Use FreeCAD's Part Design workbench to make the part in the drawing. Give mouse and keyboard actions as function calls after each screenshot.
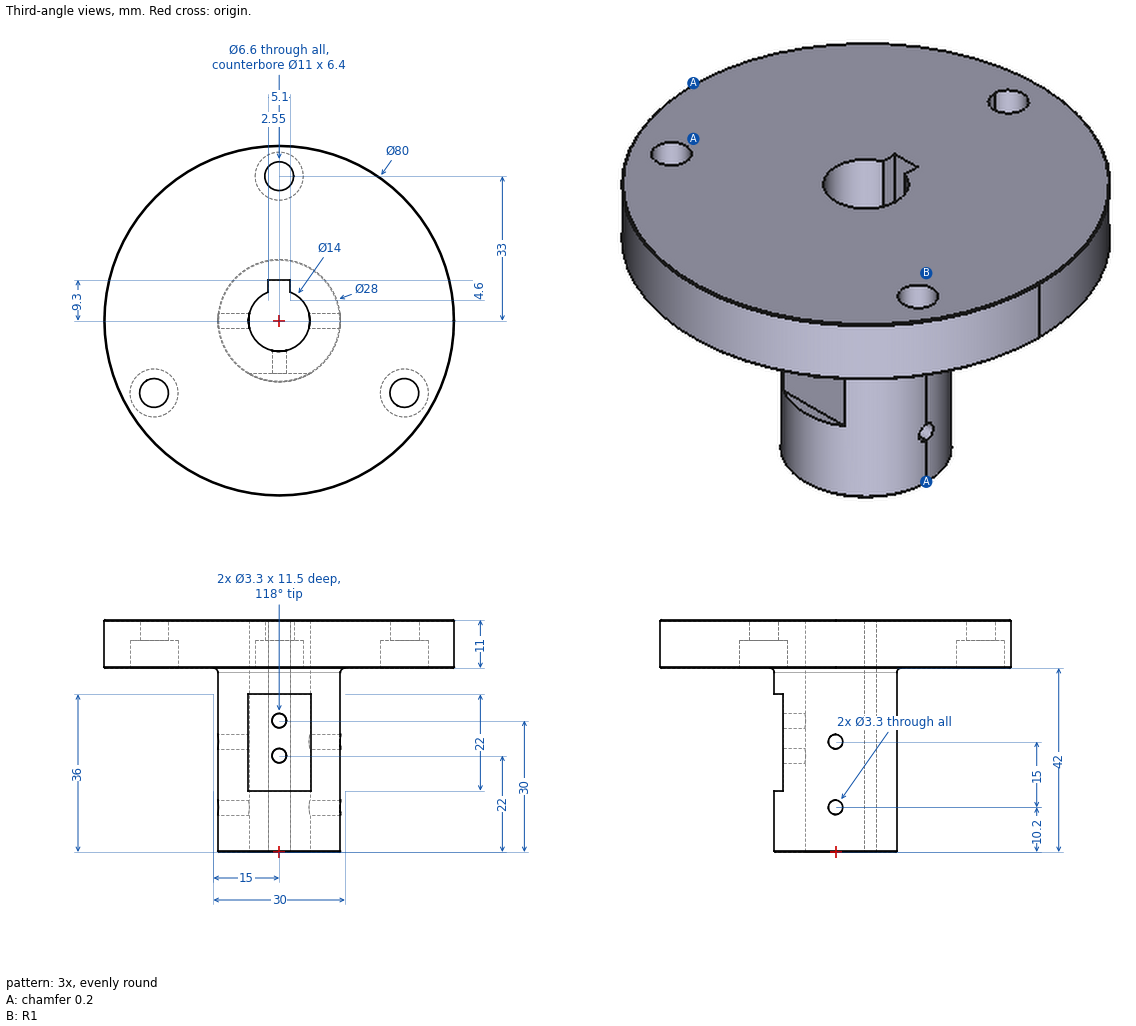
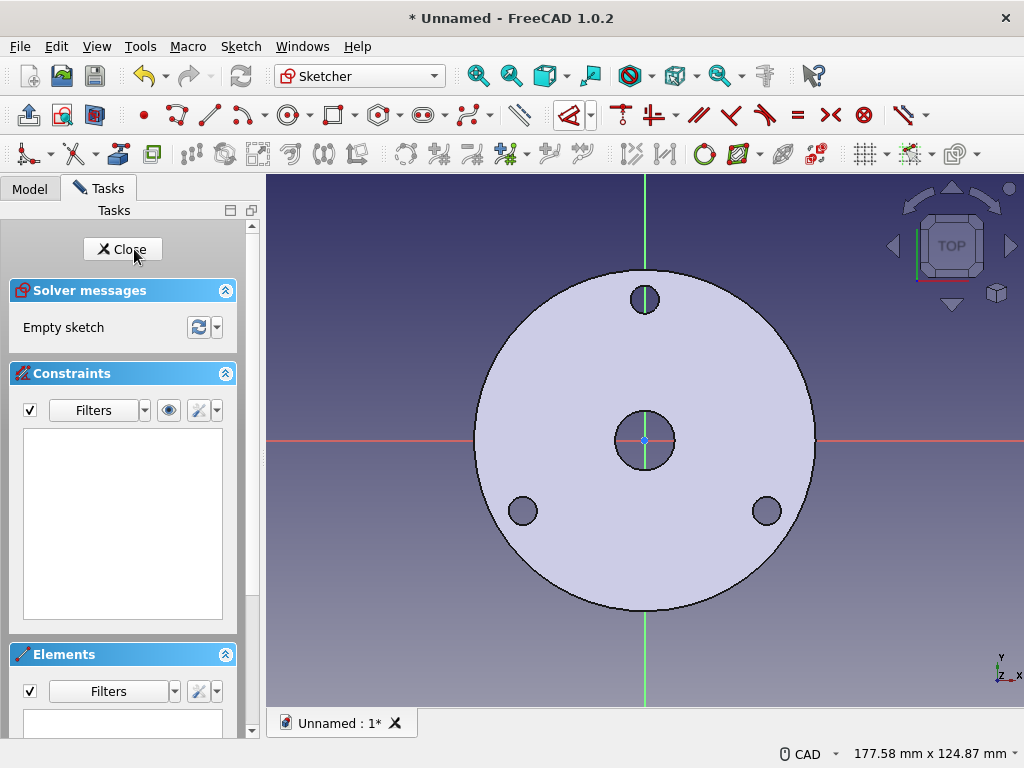
key(q)
key(s)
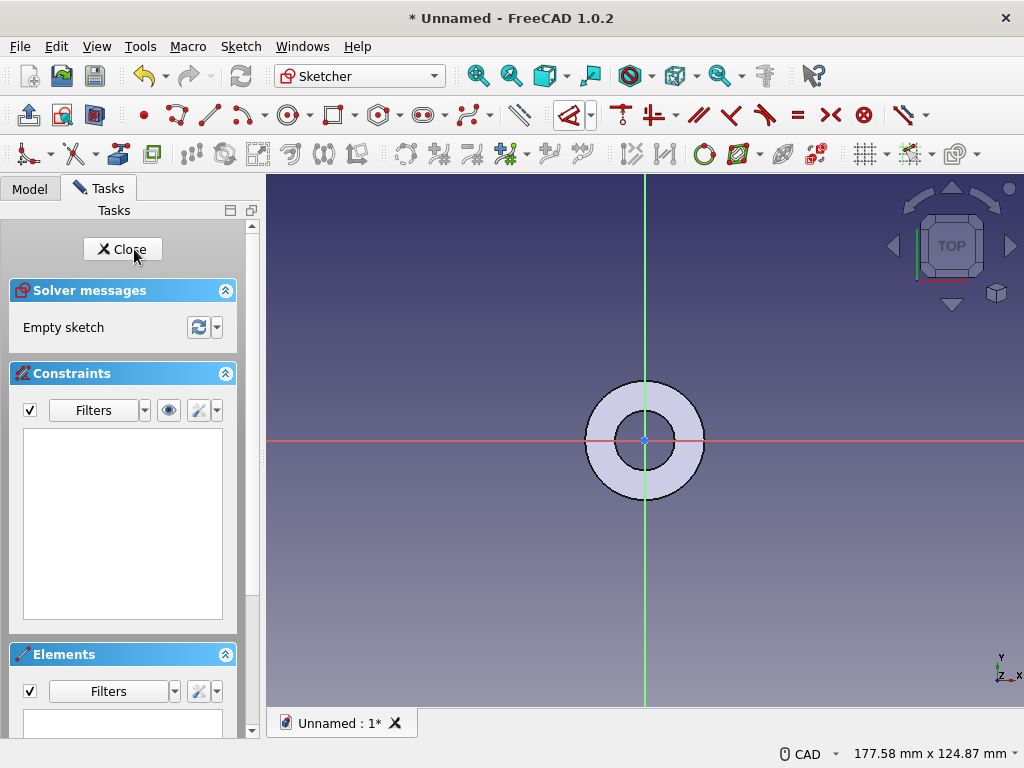
scroll(653, 418, up, 11)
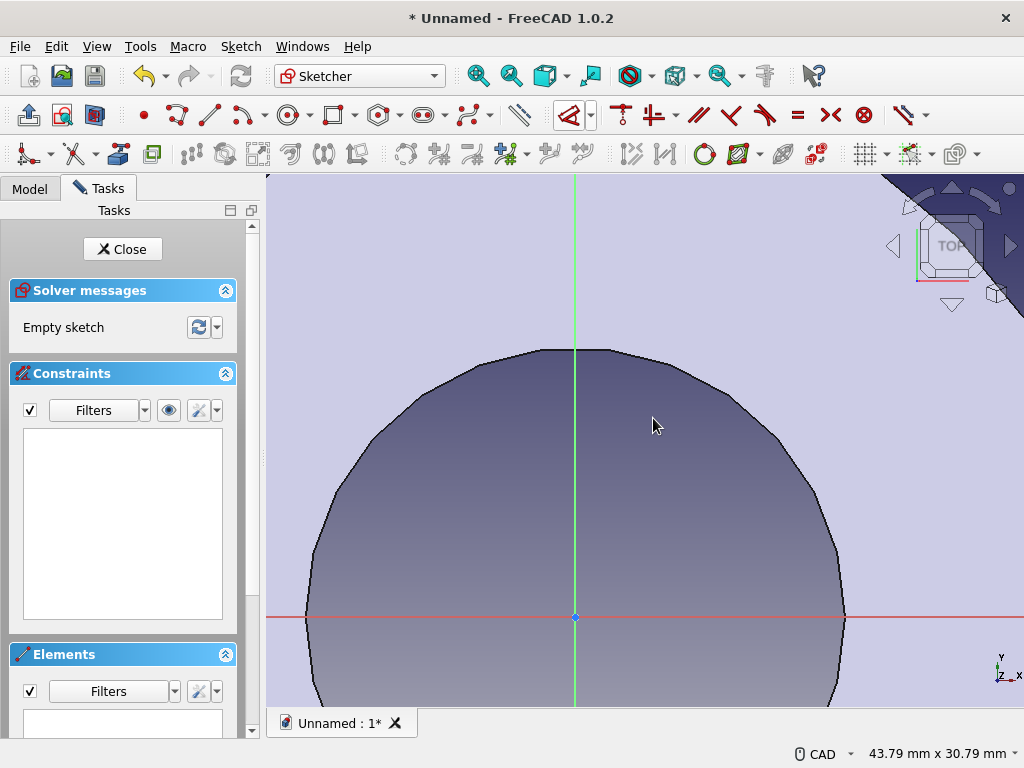
click(332, 116)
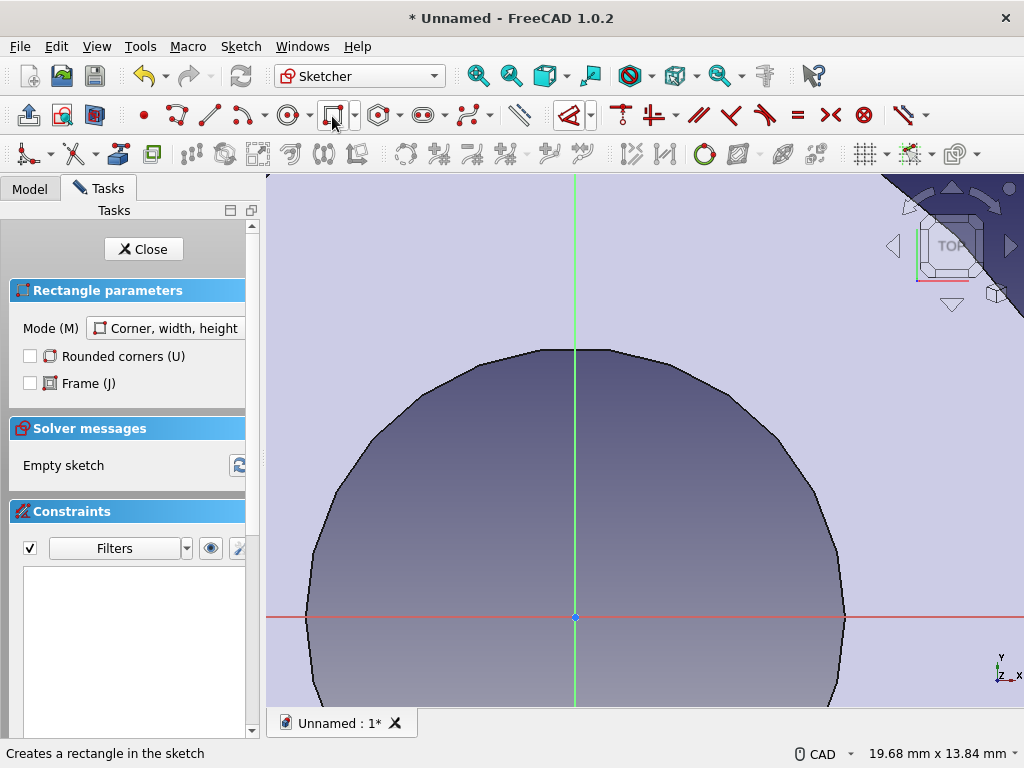
click(477, 259)
move(674, 436)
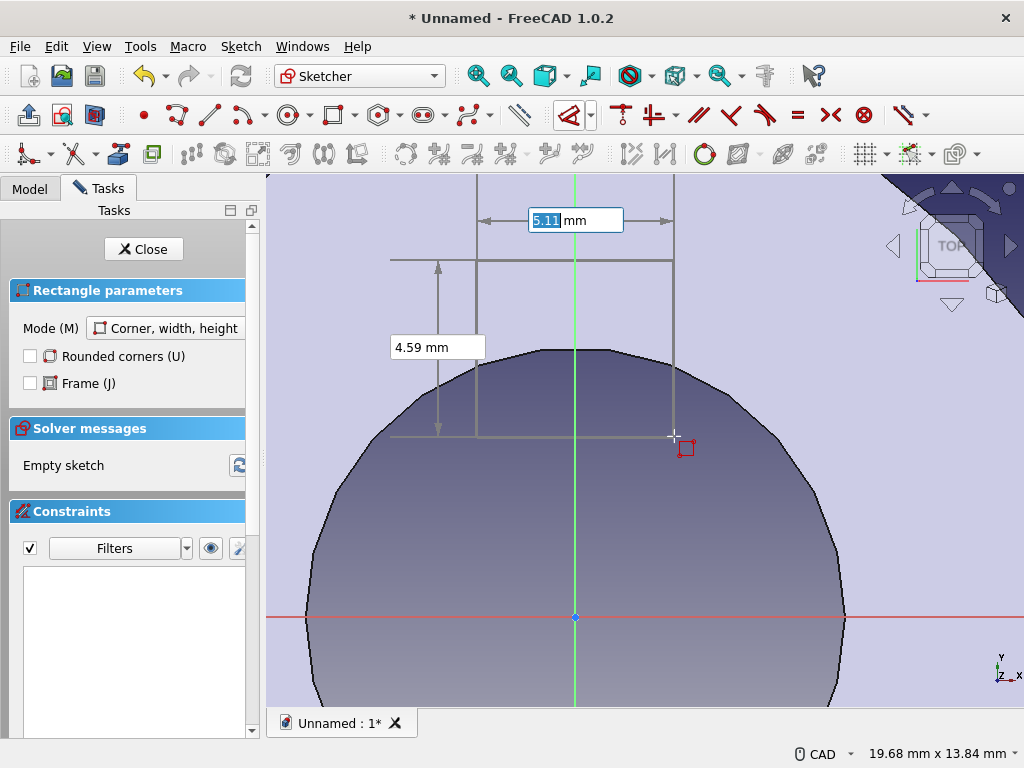
text(5.1)
key(Tab)
text(4.6)
key(Return)
key(Escape)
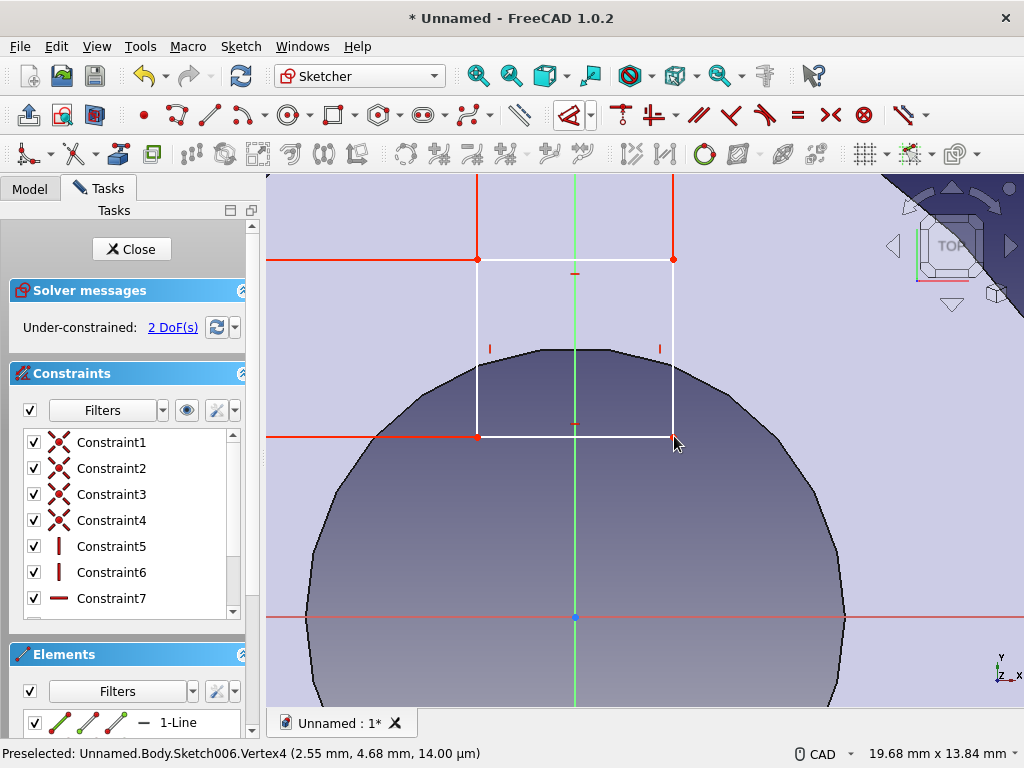
click(477, 260)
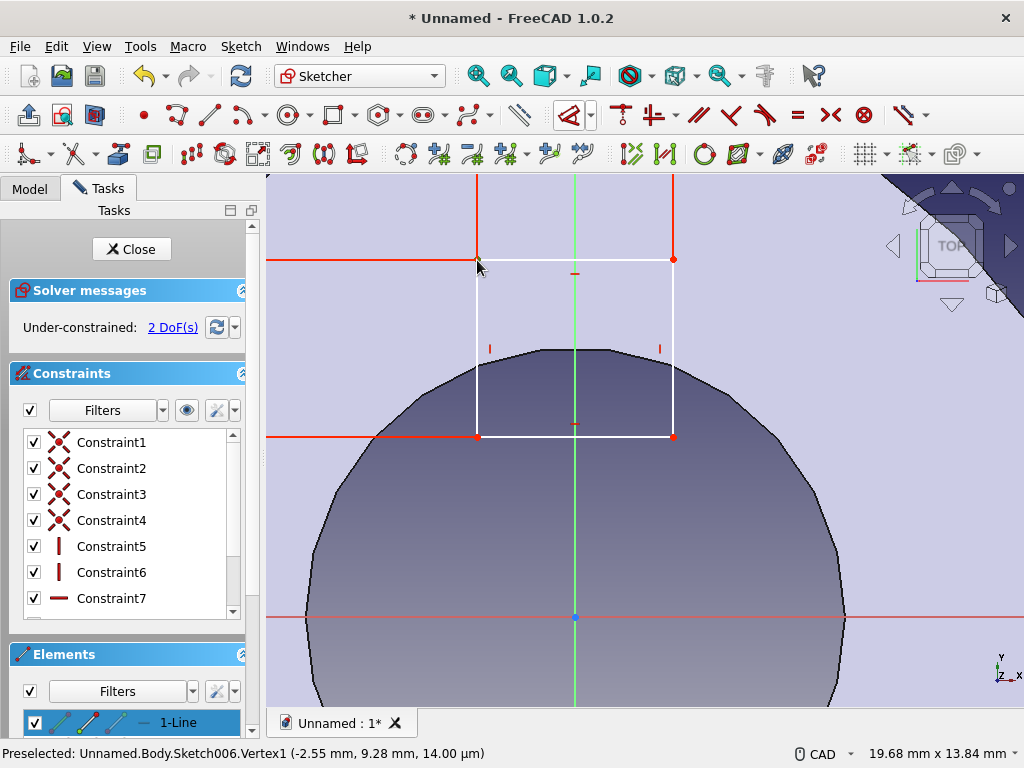
key(i)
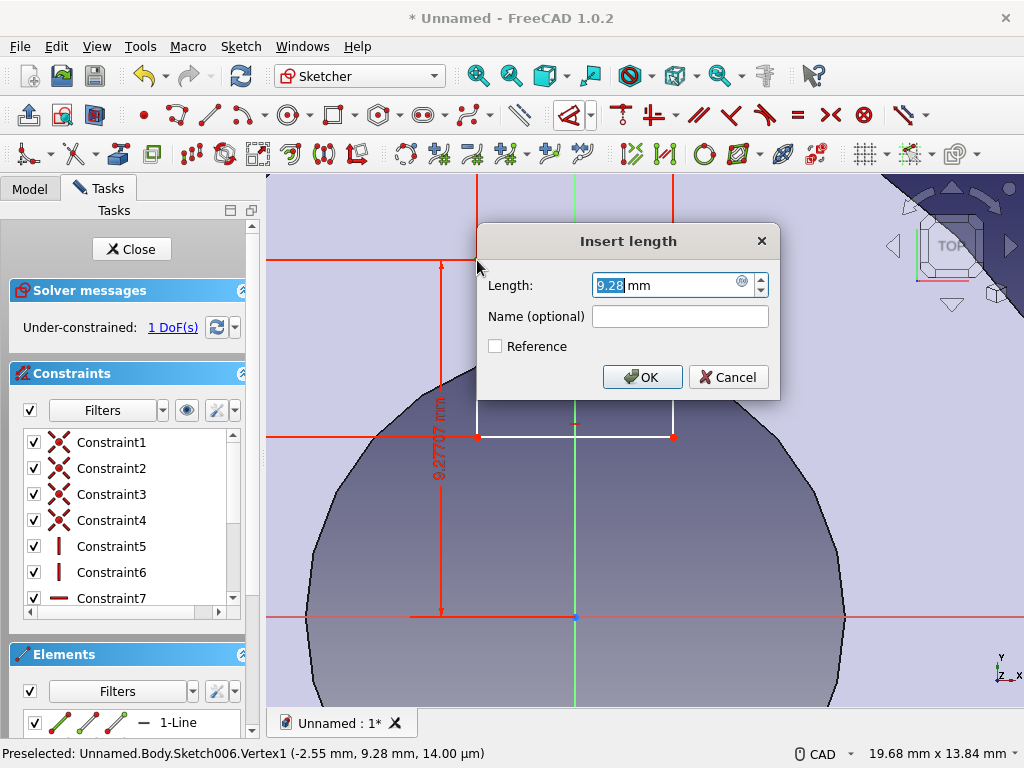
text(9.3)
key(Return)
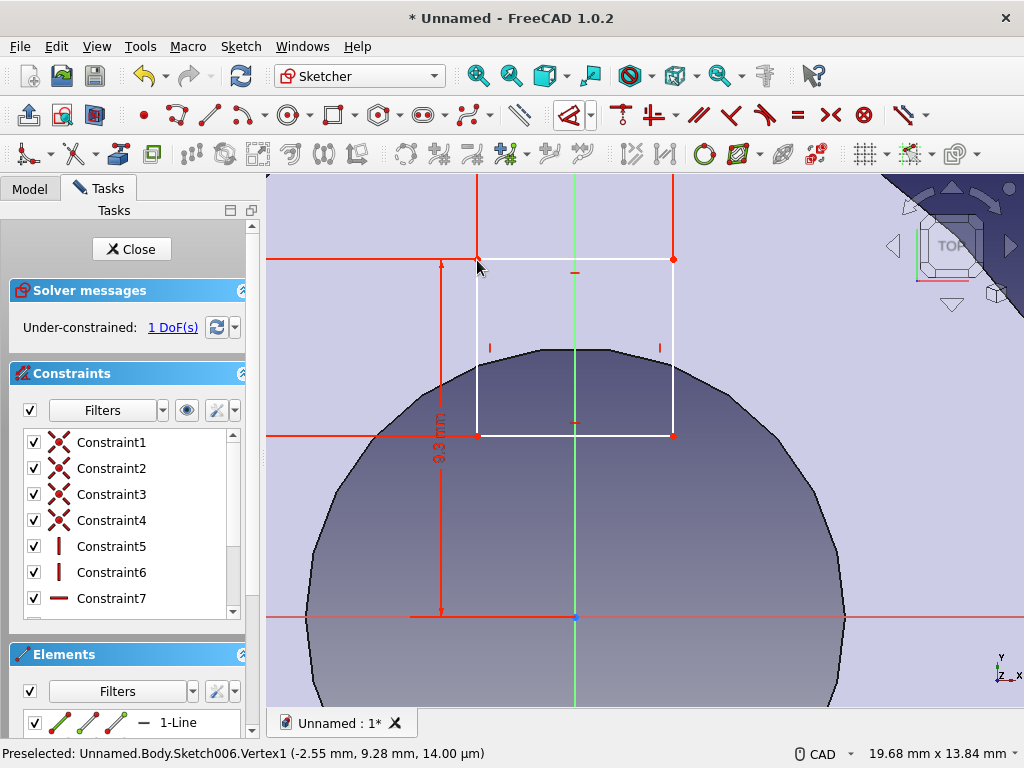
click(477, 259)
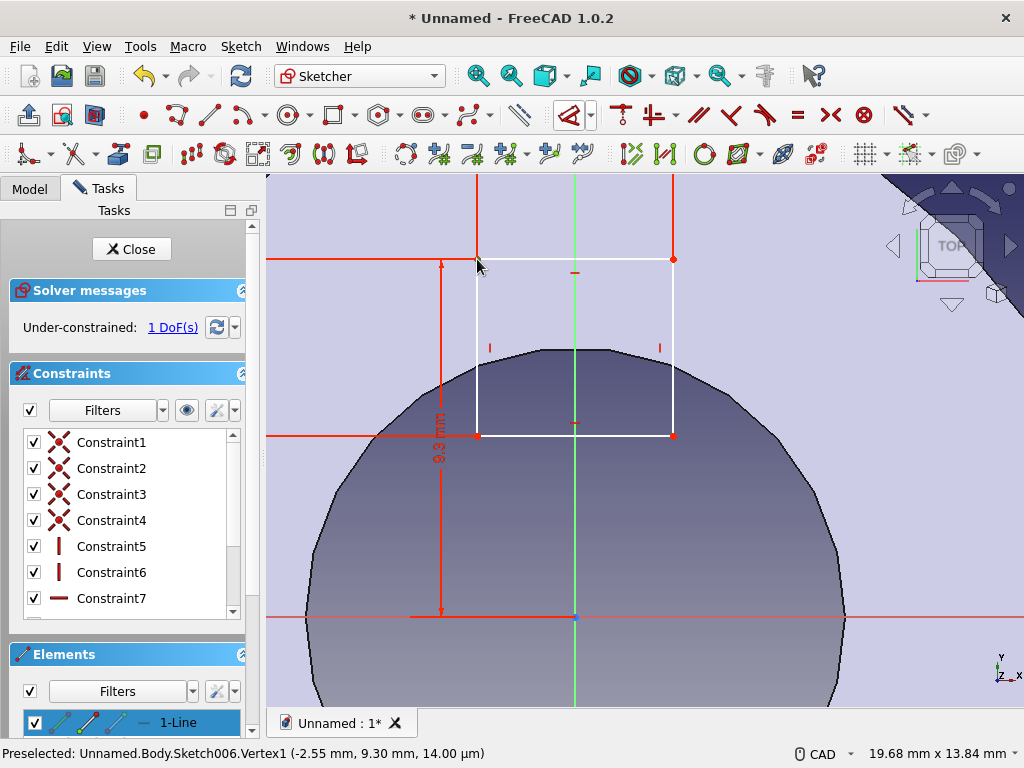
click(590, 116)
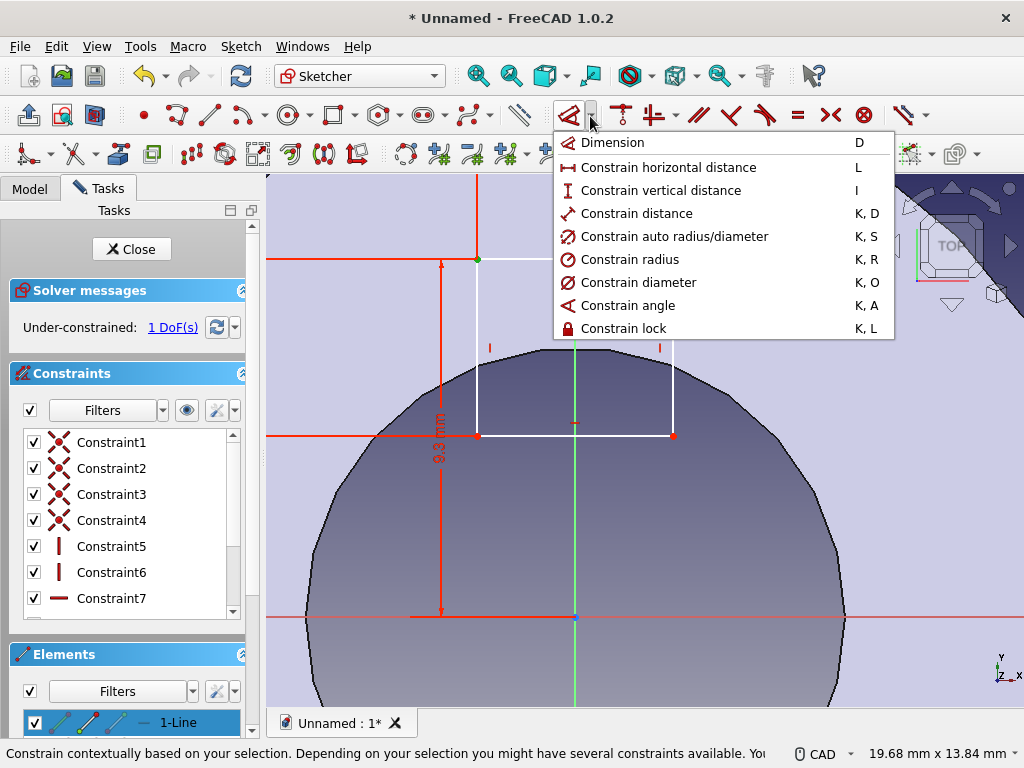
click(724, 168)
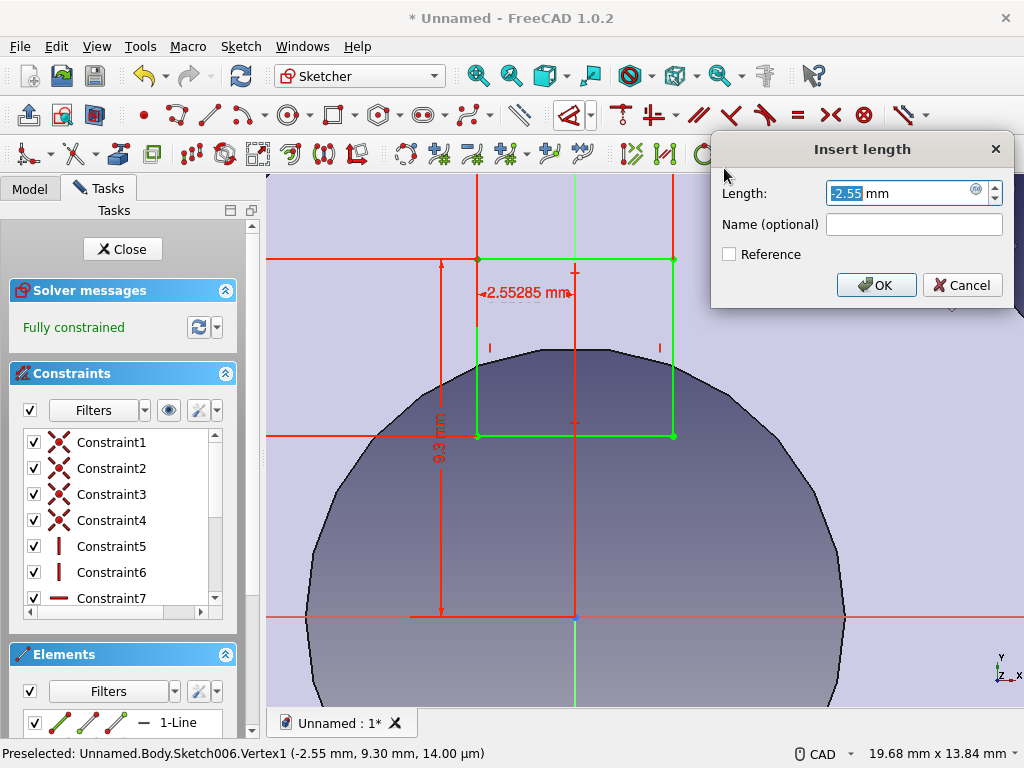
text(-2.55)
key(Return)